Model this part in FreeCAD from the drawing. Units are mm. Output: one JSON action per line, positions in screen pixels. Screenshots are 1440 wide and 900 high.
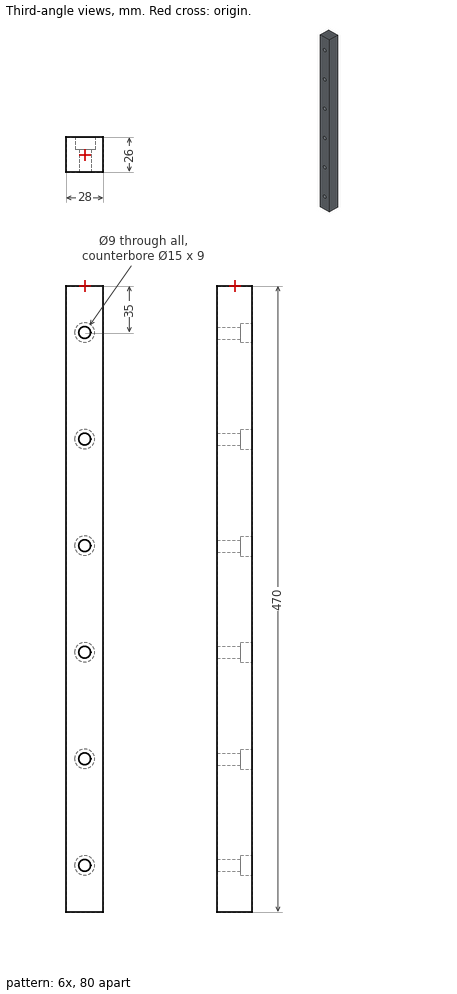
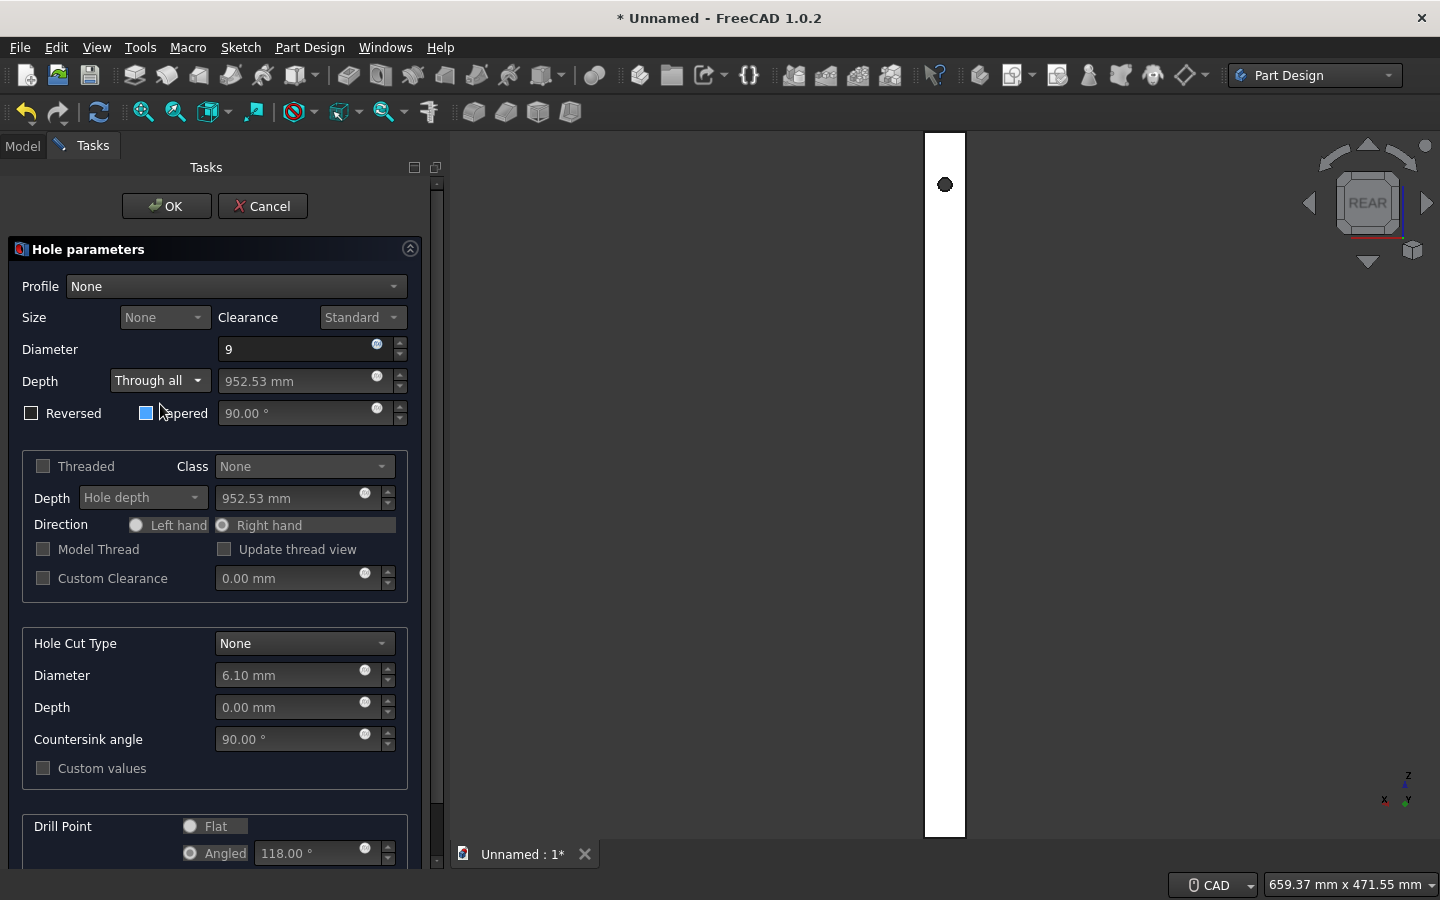
{"action": "left_click", "coordinate": [306, 644]}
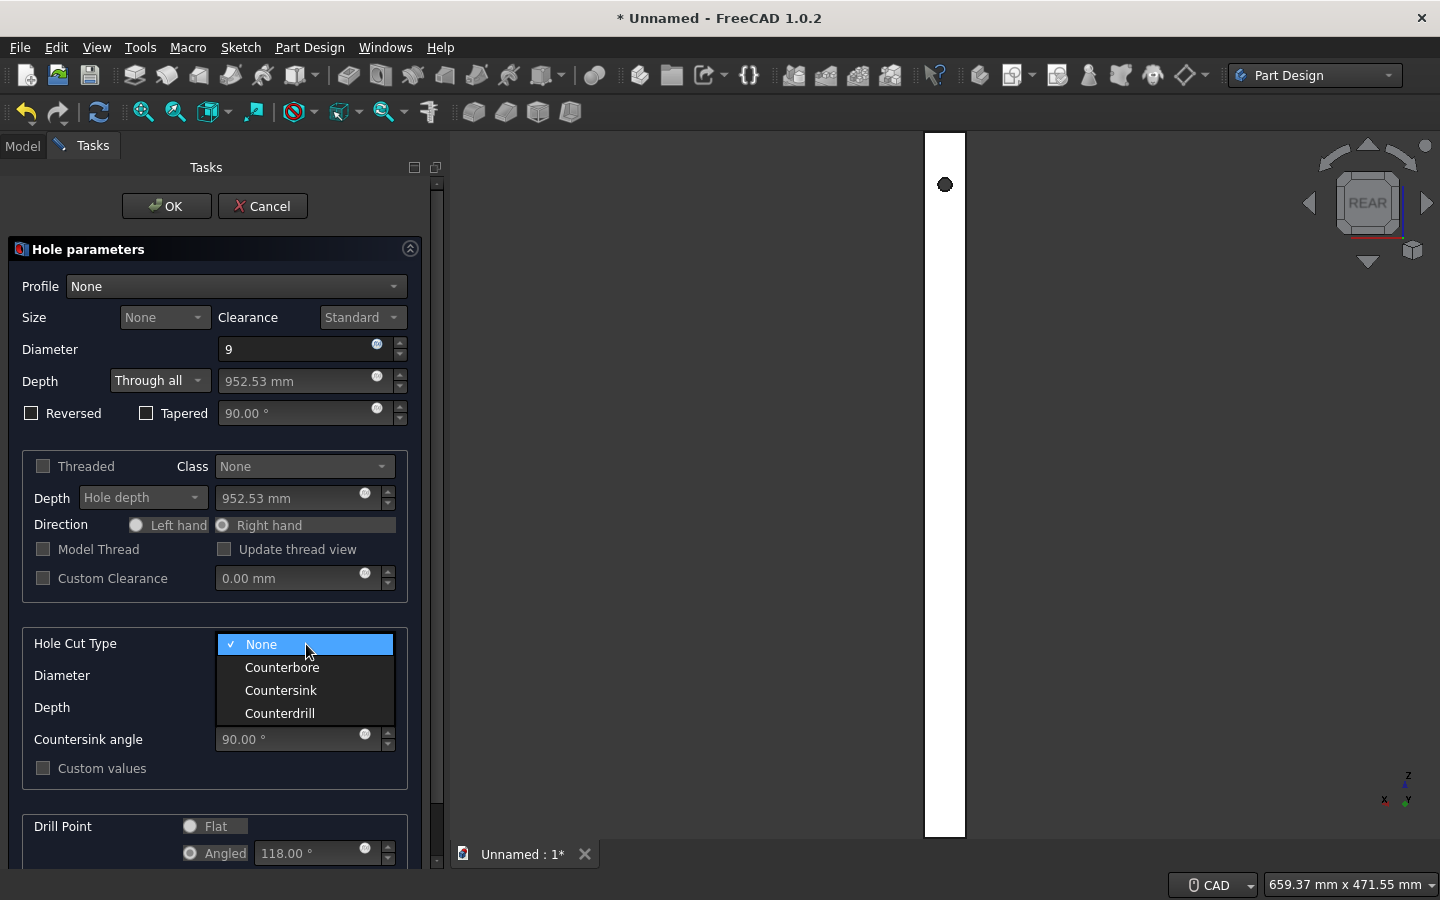
{"action": "left_click", "coordinate": [304, 668]}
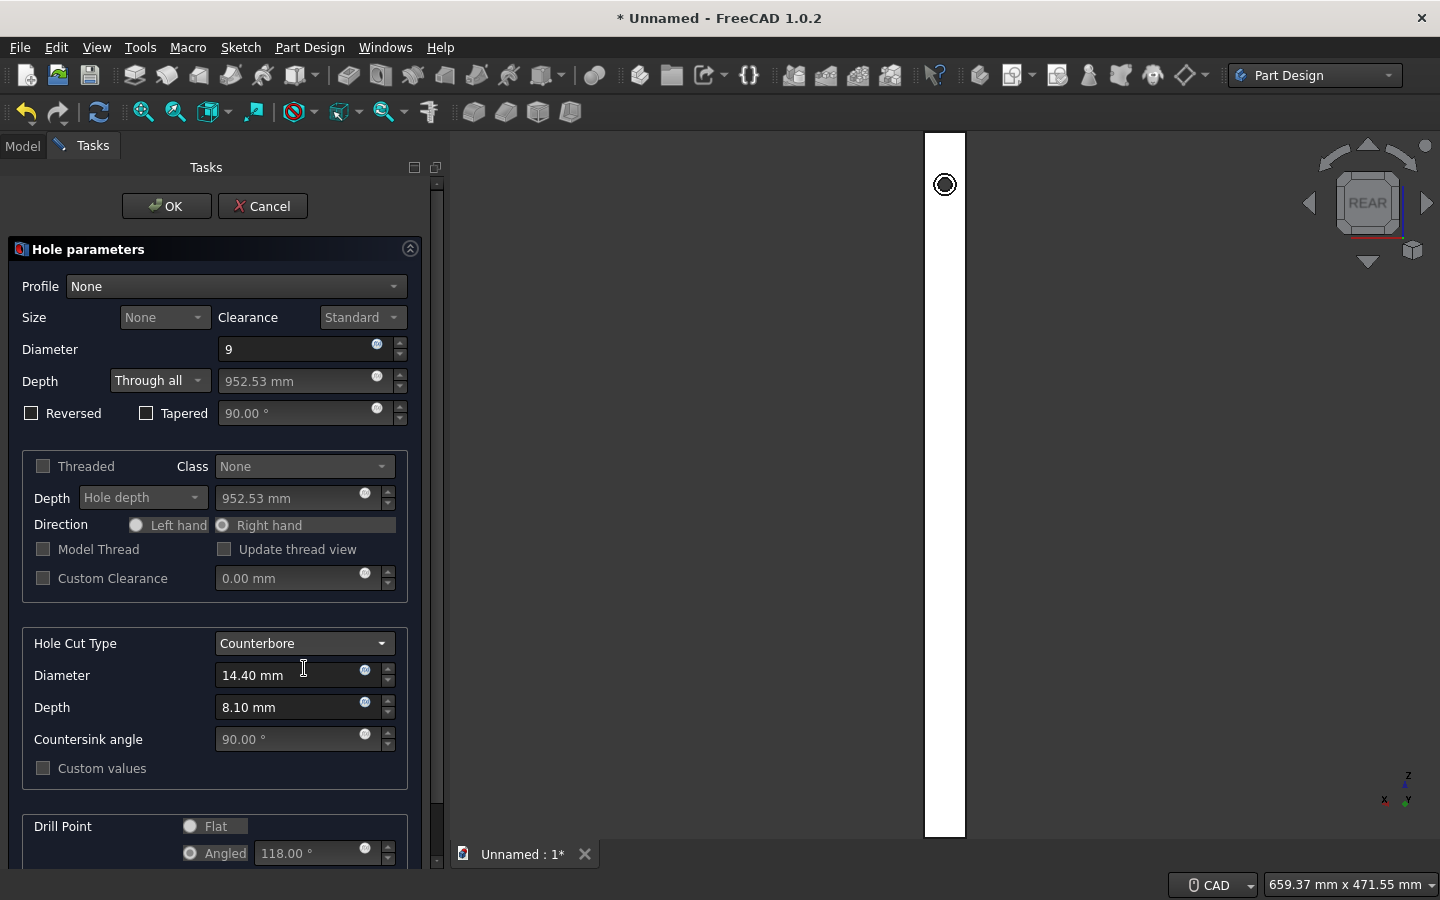
{"action": "triple_click", "coordinate": [298, 675]}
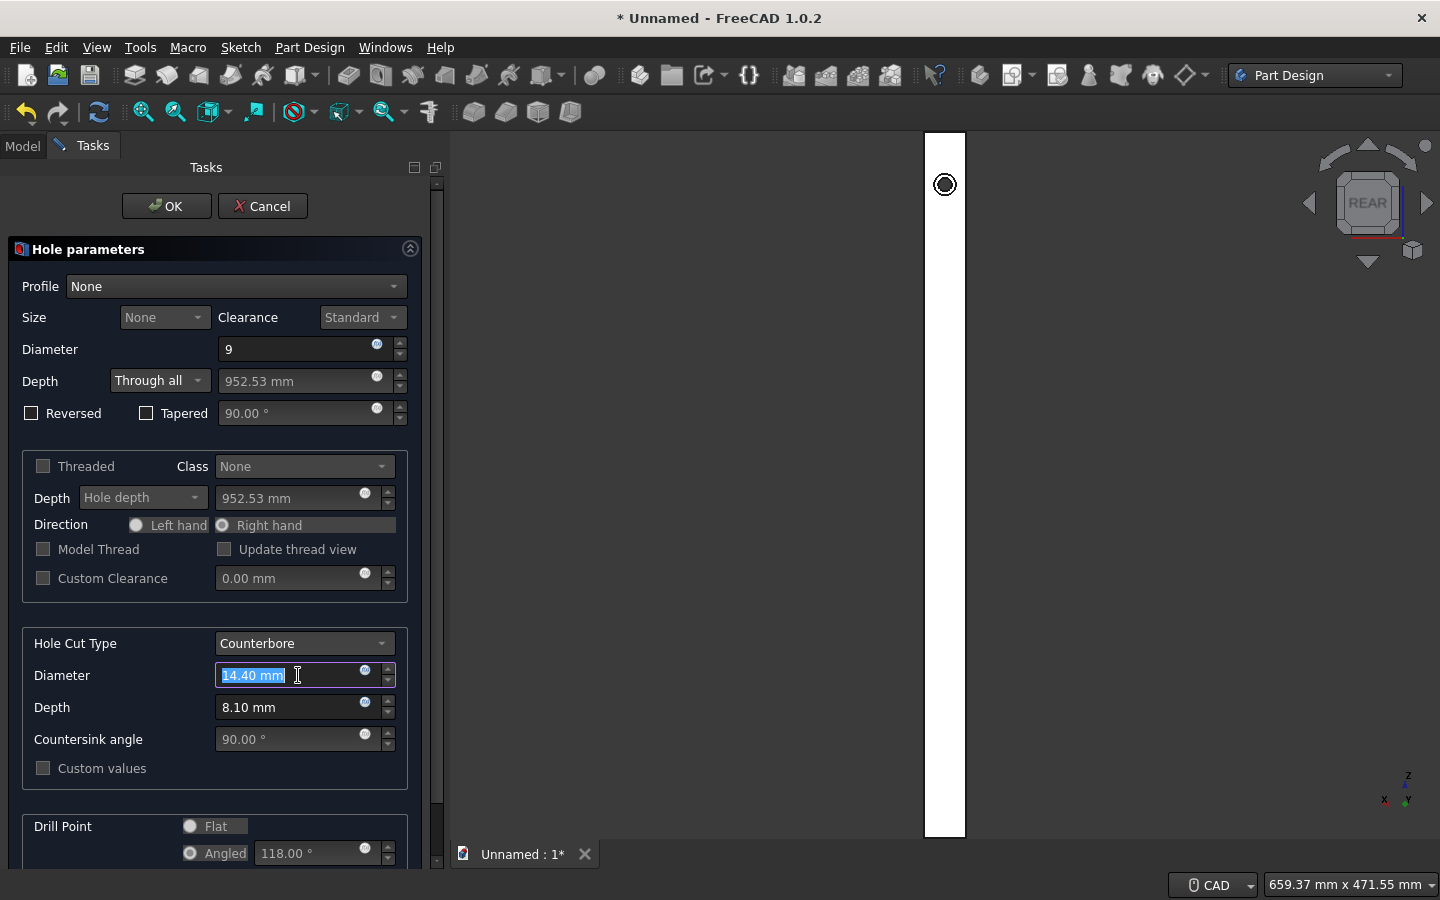
{"action": "type", "text": "15"}
{"action": "key", "text": "Tab"}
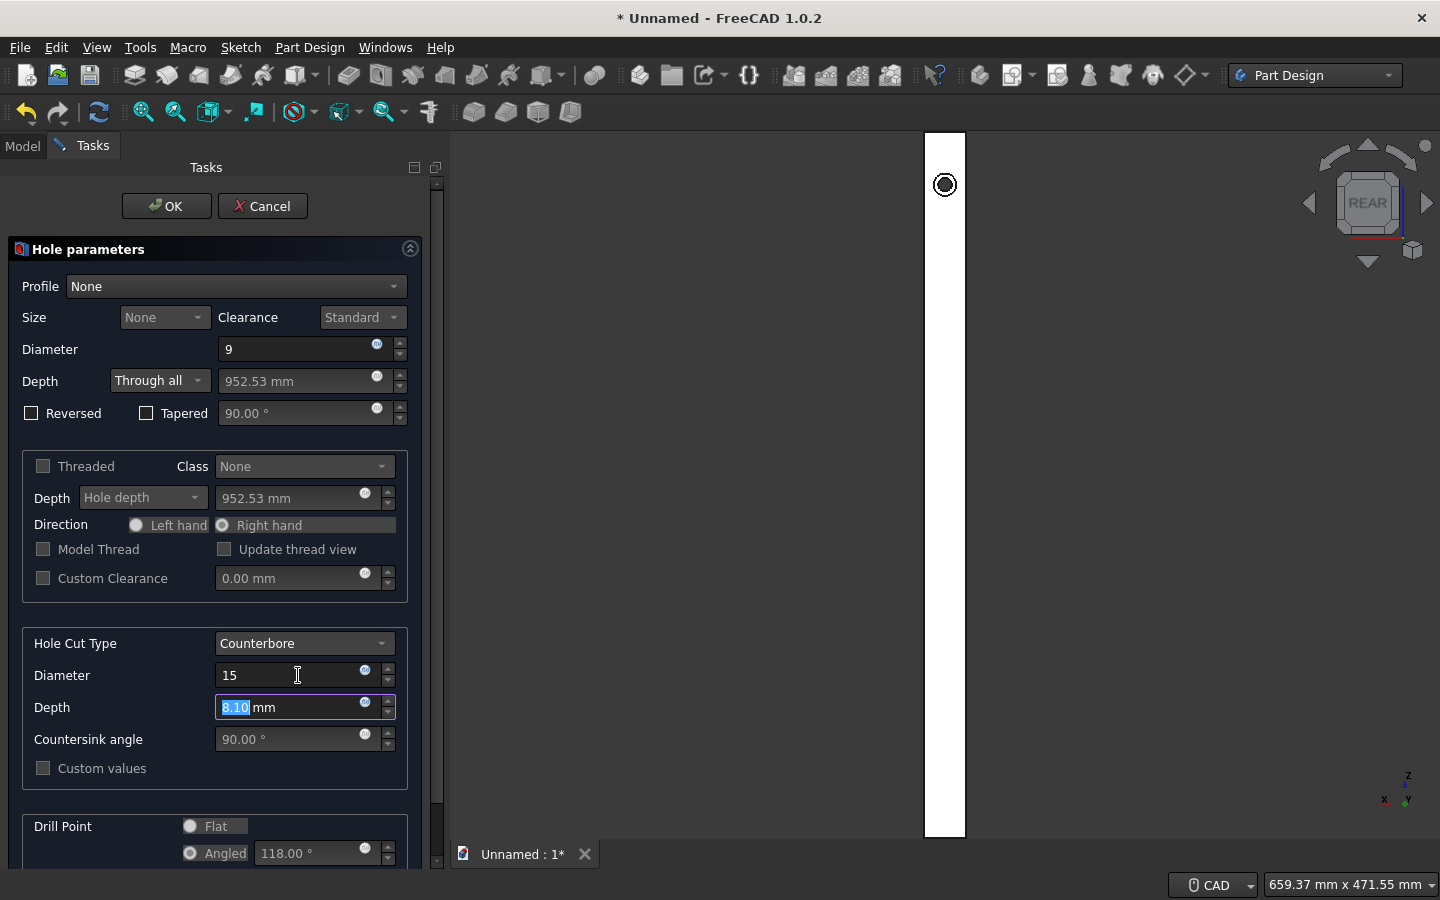
{"action": "type", "text": "9"}
{"action": "key", "text": "Tab"}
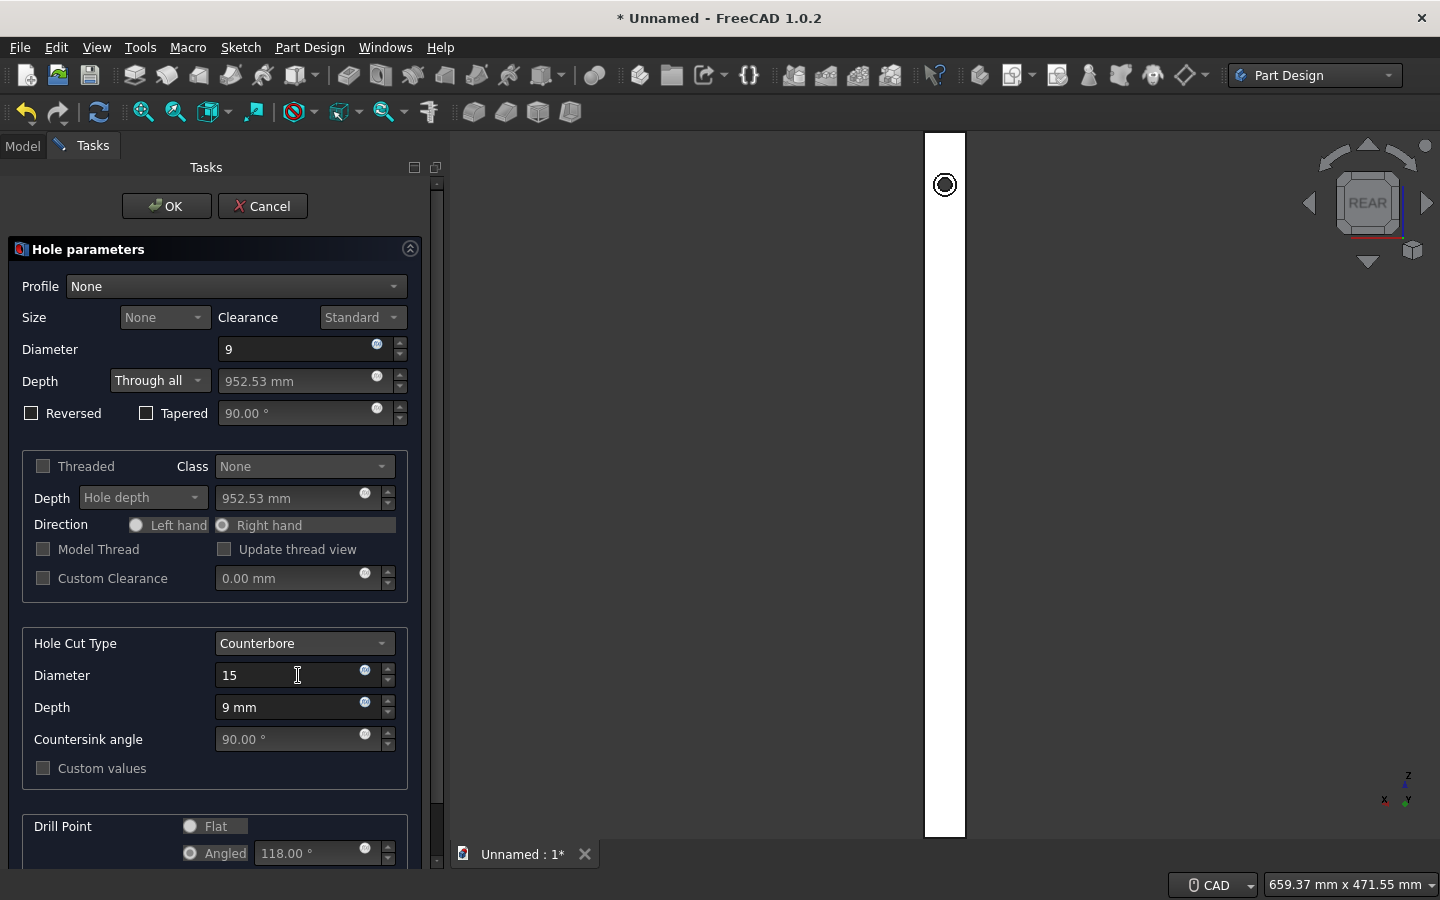
{"action": "left_click", "coordinate": [167, 206]}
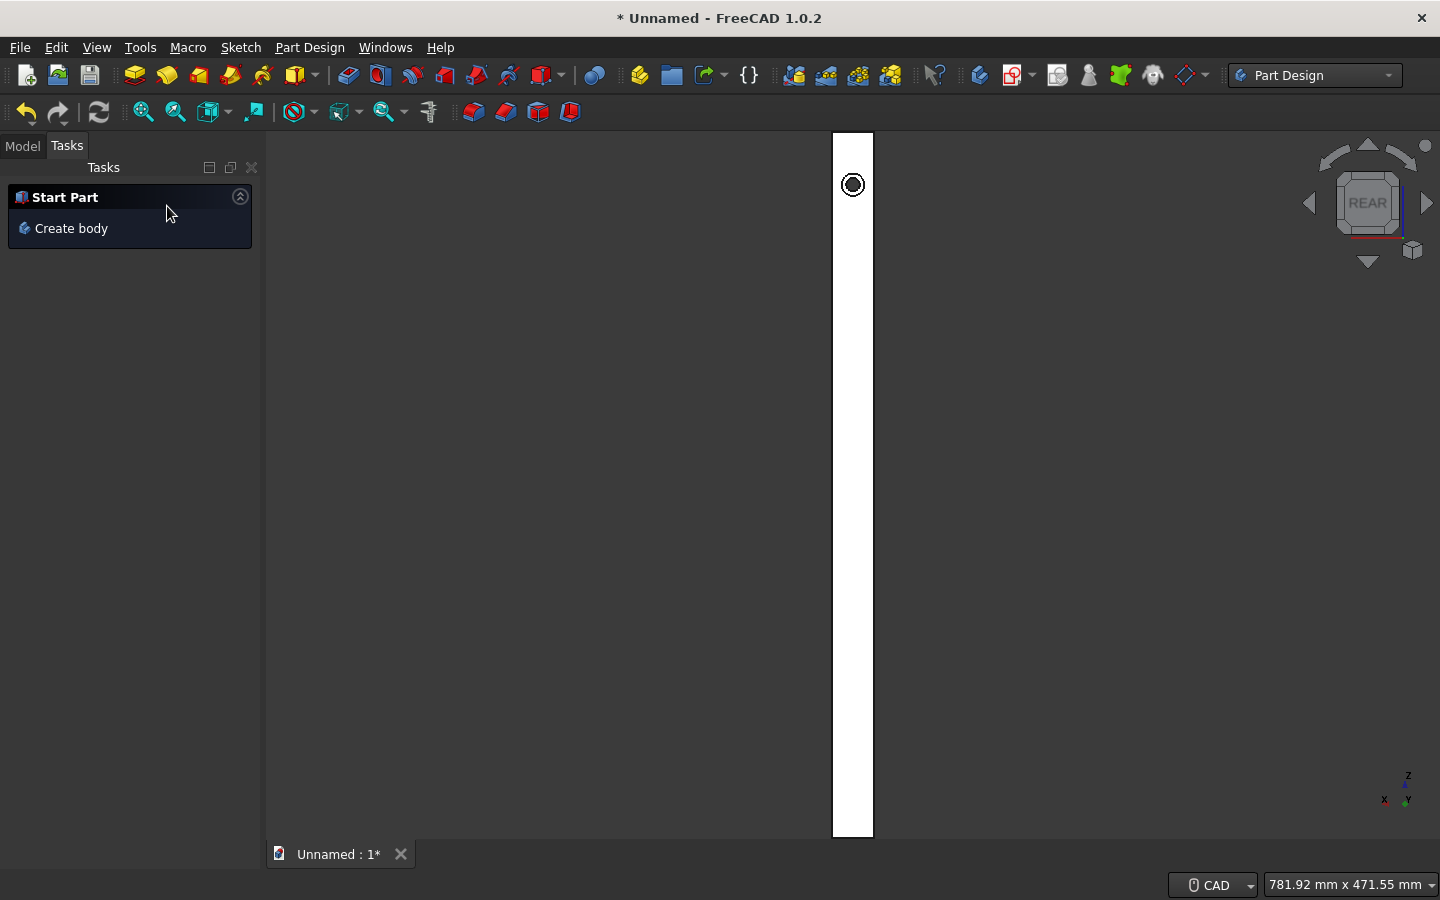
{"action": "left_click", "coordinate": [23, 145]}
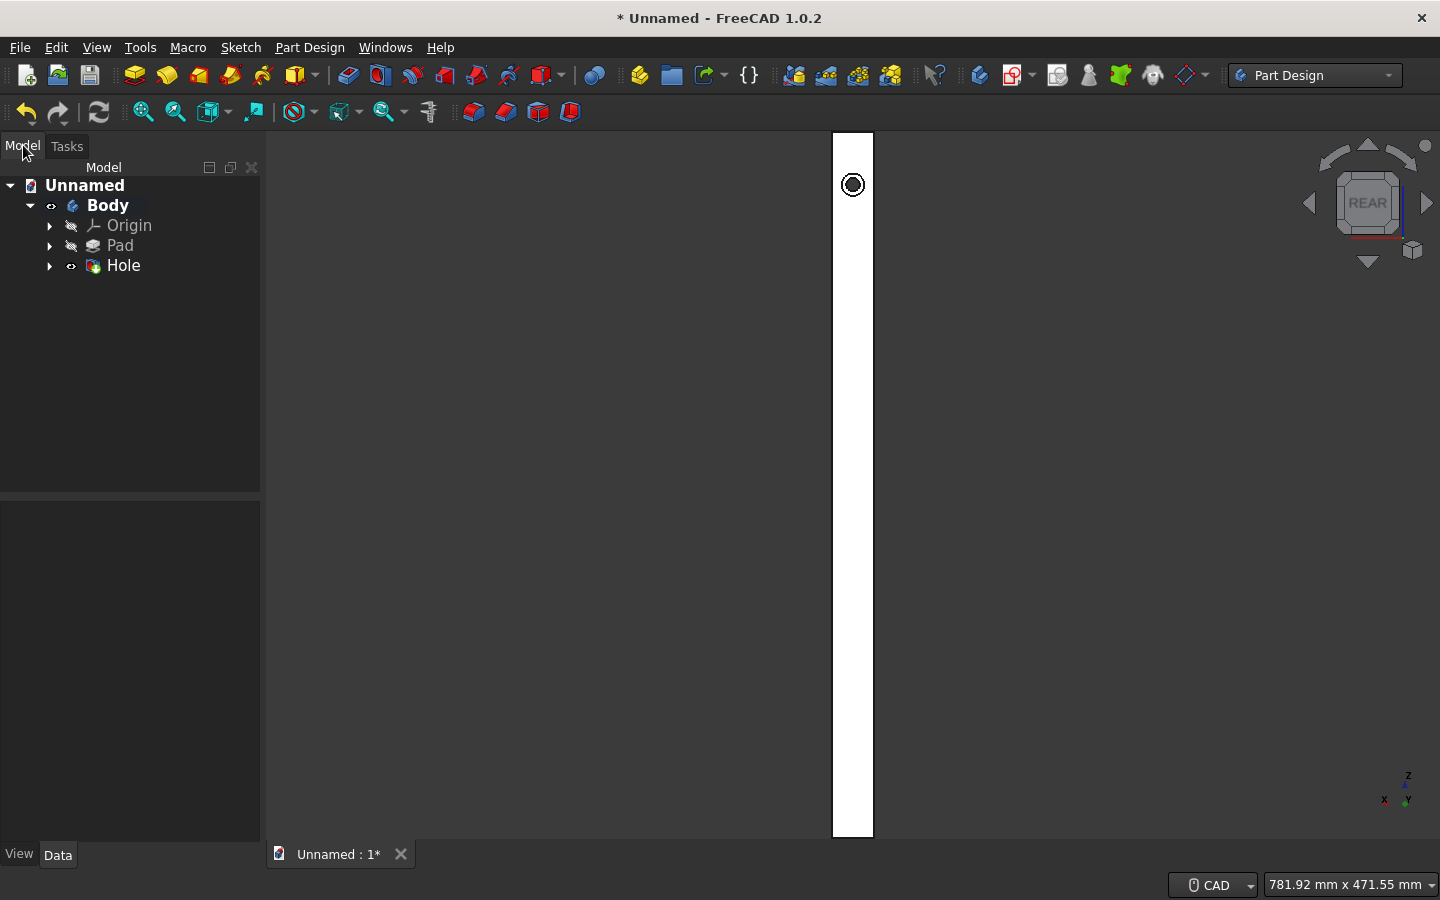
{"action": "left_click", "coordinate": [116, 266]}